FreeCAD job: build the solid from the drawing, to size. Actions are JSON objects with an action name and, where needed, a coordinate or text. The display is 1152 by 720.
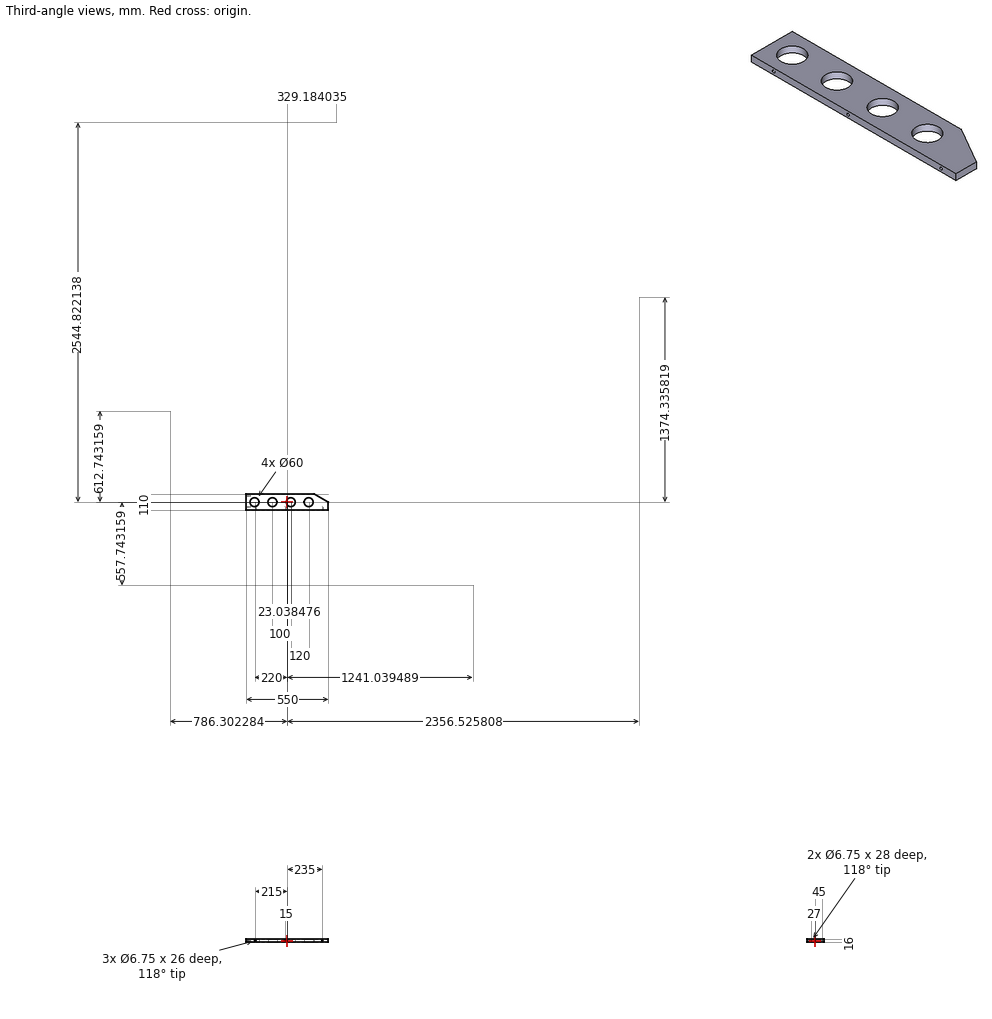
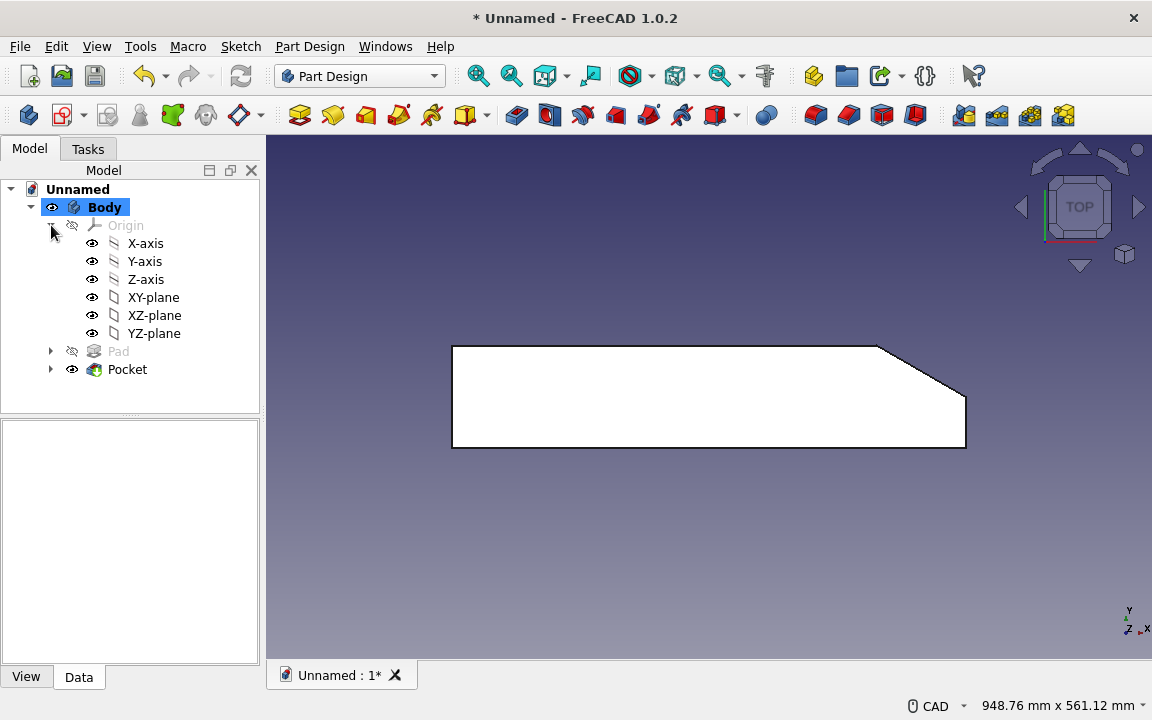
{"action": "left_click", "coordinate": [137, 315]}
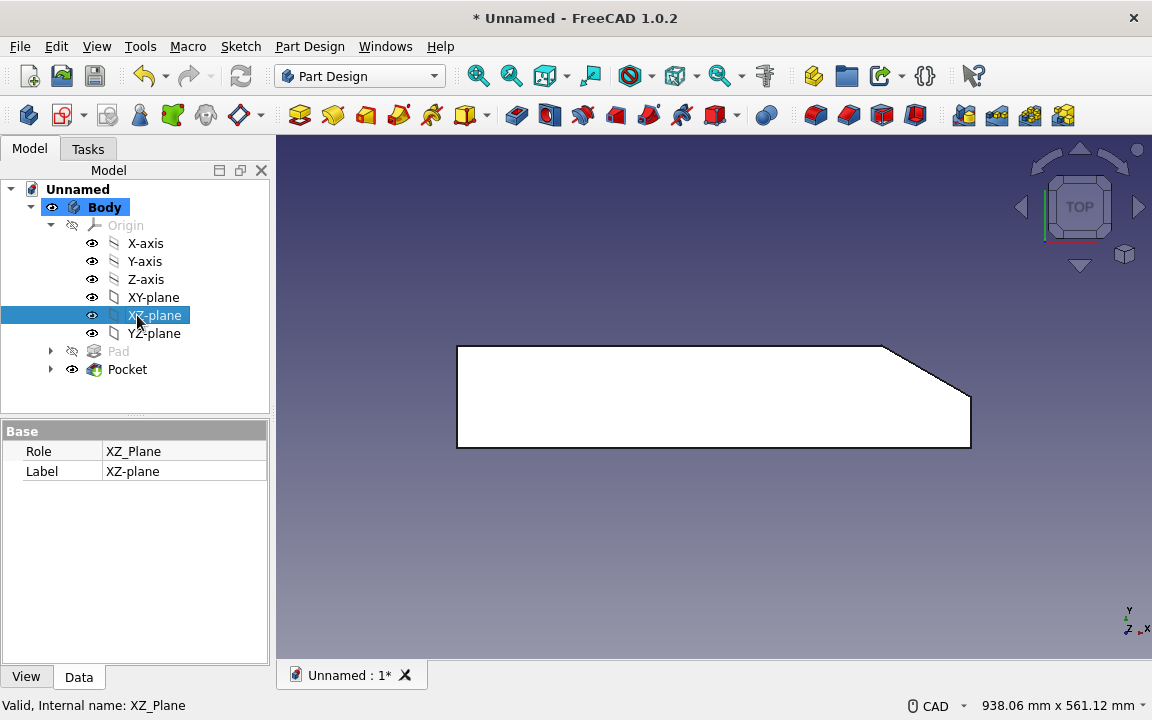
{"action": "left_click", "coordinate": [238, 116]}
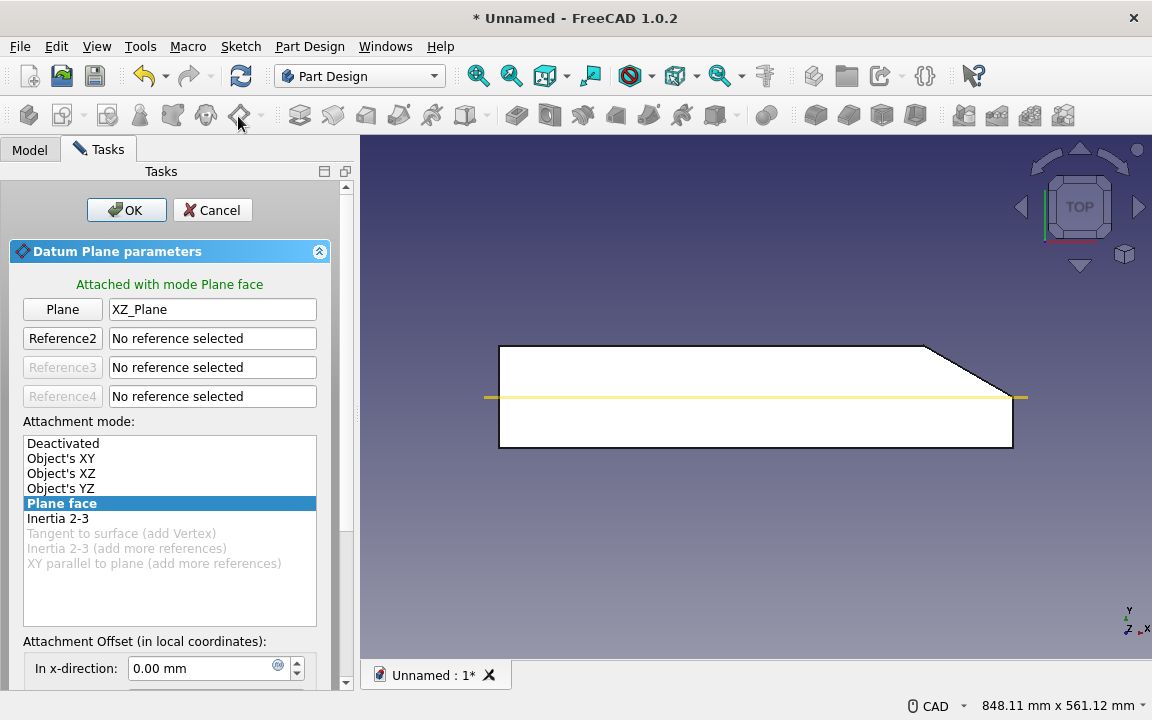
{"action": "scroll", "coordinate": [346, 436], "scroll_direction": "down", "scroll_amount": 2}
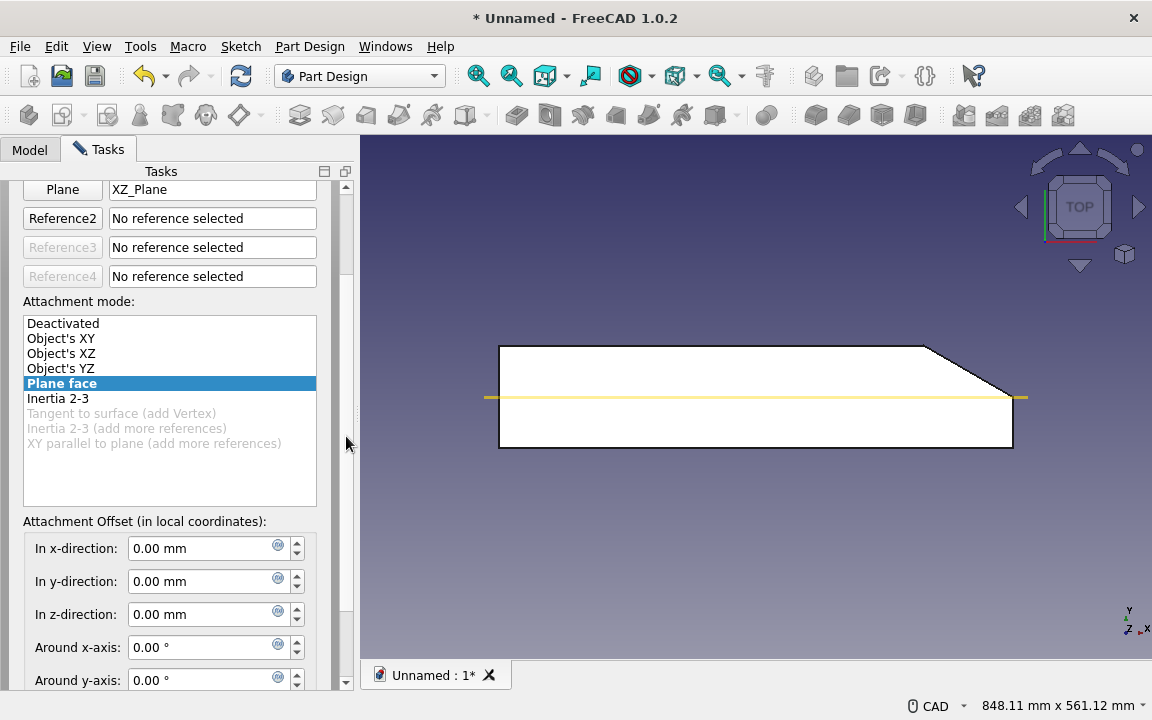
{"action": "triple_click", "coordinate": [210, 614]}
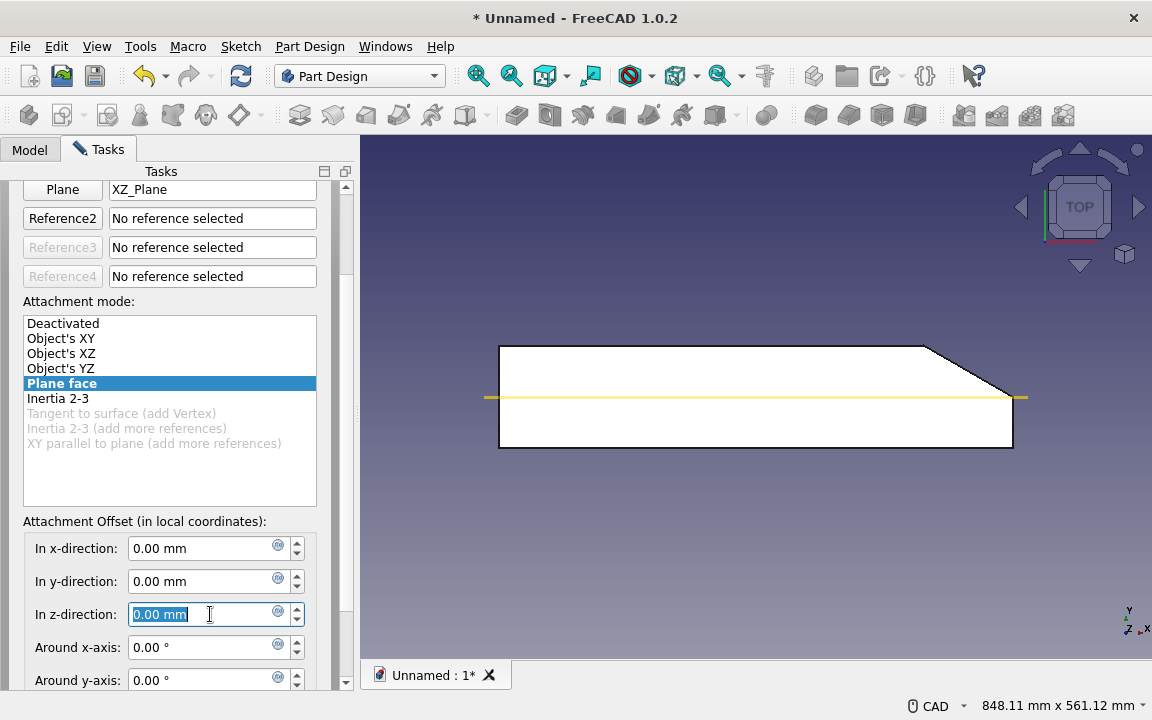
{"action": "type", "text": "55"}
{"action": "key", "text": "Tab"}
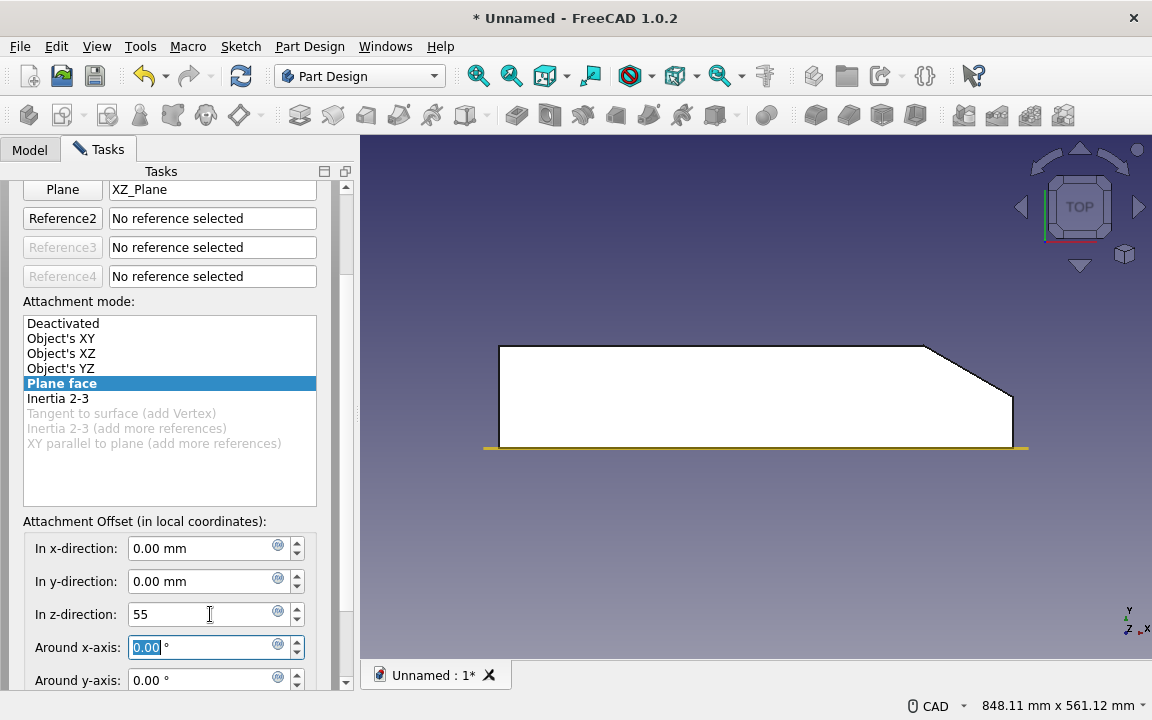
{"action": "scroll", "coordinate": [346, 436], "scroll_direction": "up", "scroll_amount": 3}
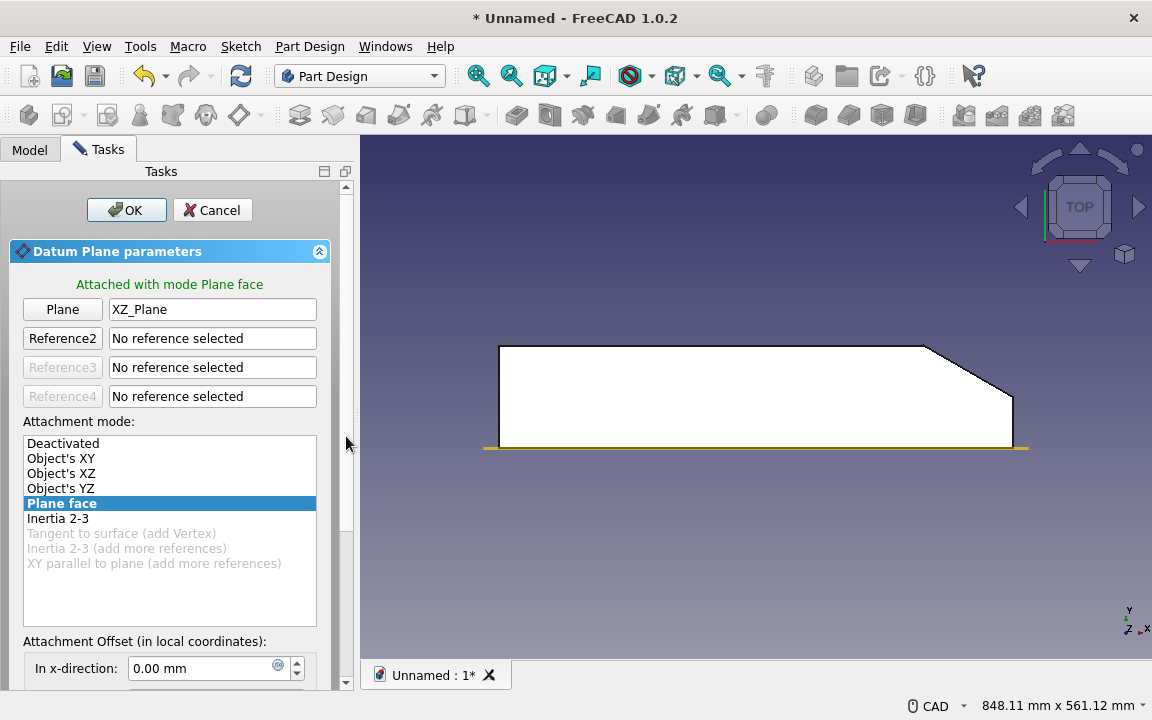
{"action": "left_click", "coordinate": [127, 210]}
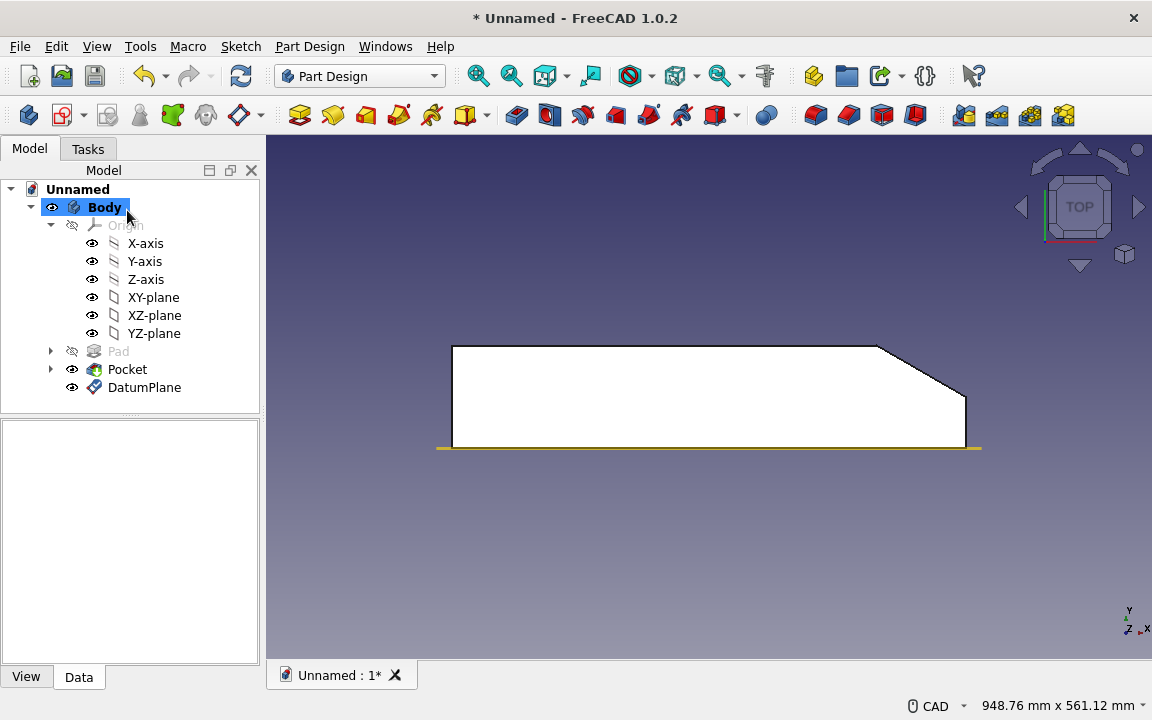
{"action": "left_click", "coordinate": [117, 387]}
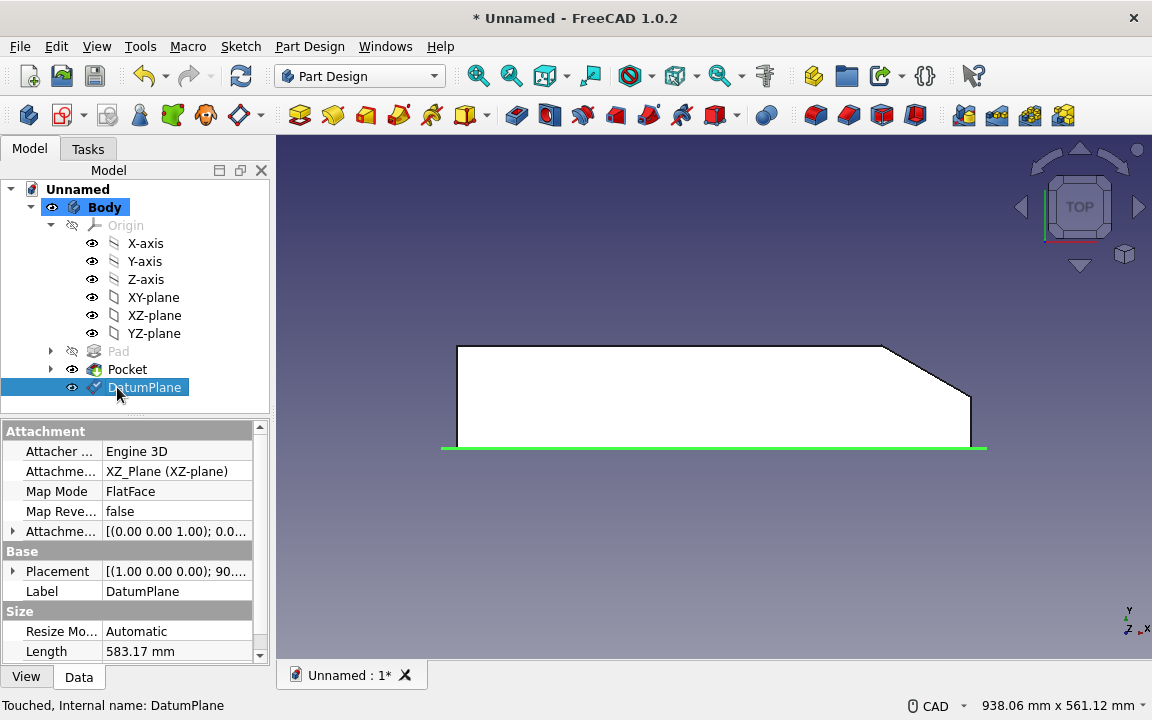
{"action": "left_click", "coordinate": [62, 116]}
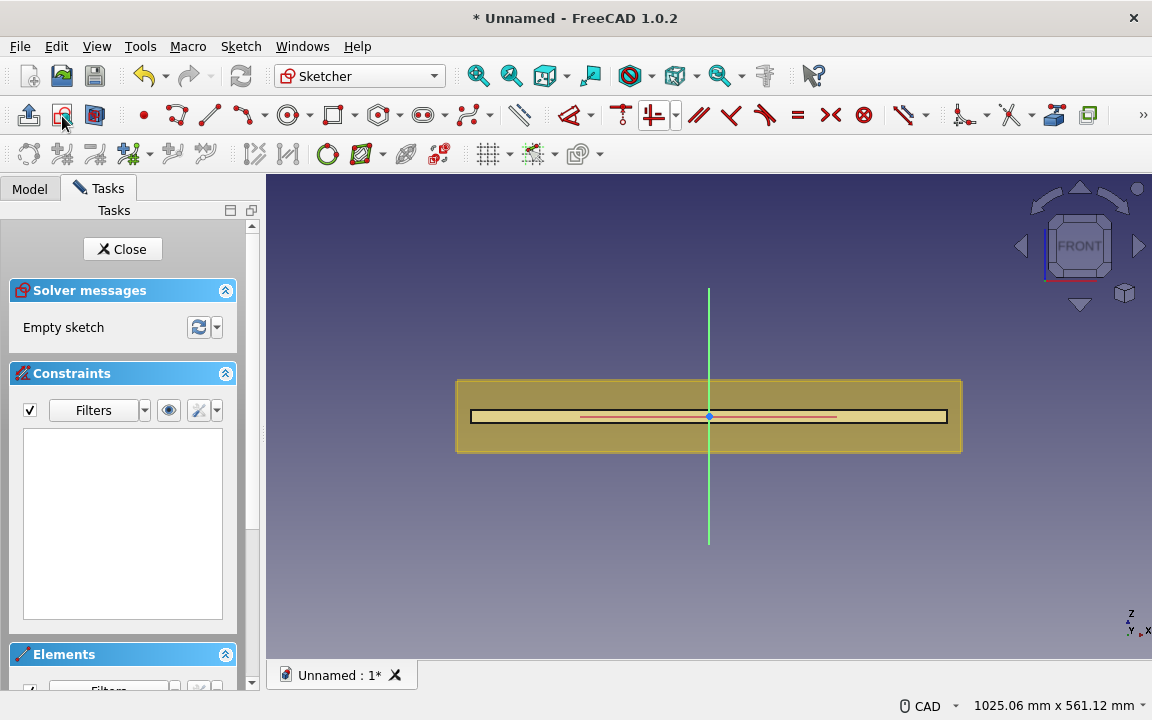
{"action": "left_click", "coordinate": [288, 116]}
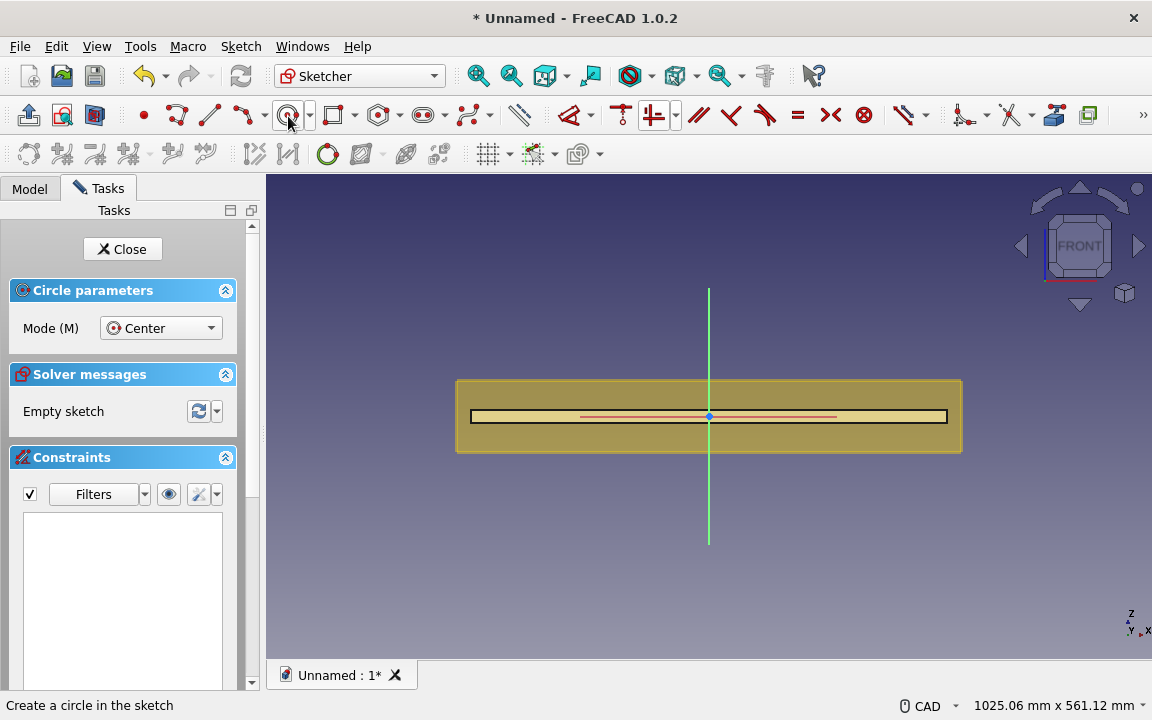
{"action": "scroll", "coordinate": [523, 416], "scroll_direction": "up", "scroll_amount": 11}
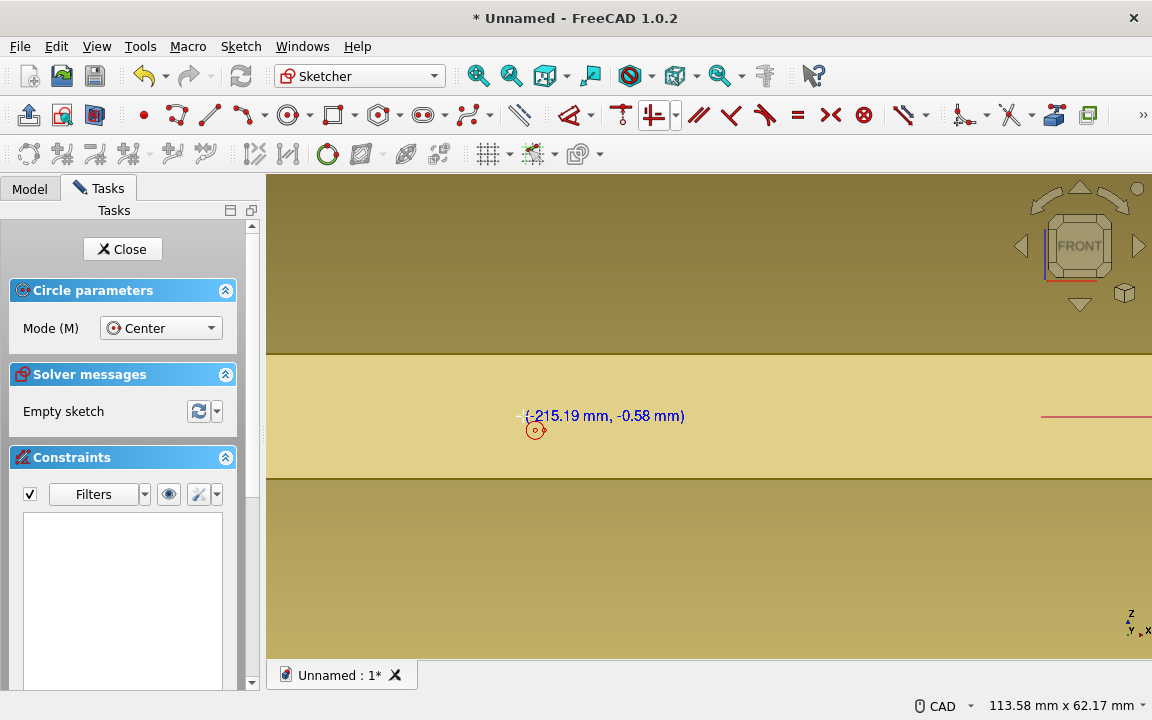
{"action": "scroll", "coordinate": [384, 417], "scroll_direction": "down", "scroll_amount": 10}